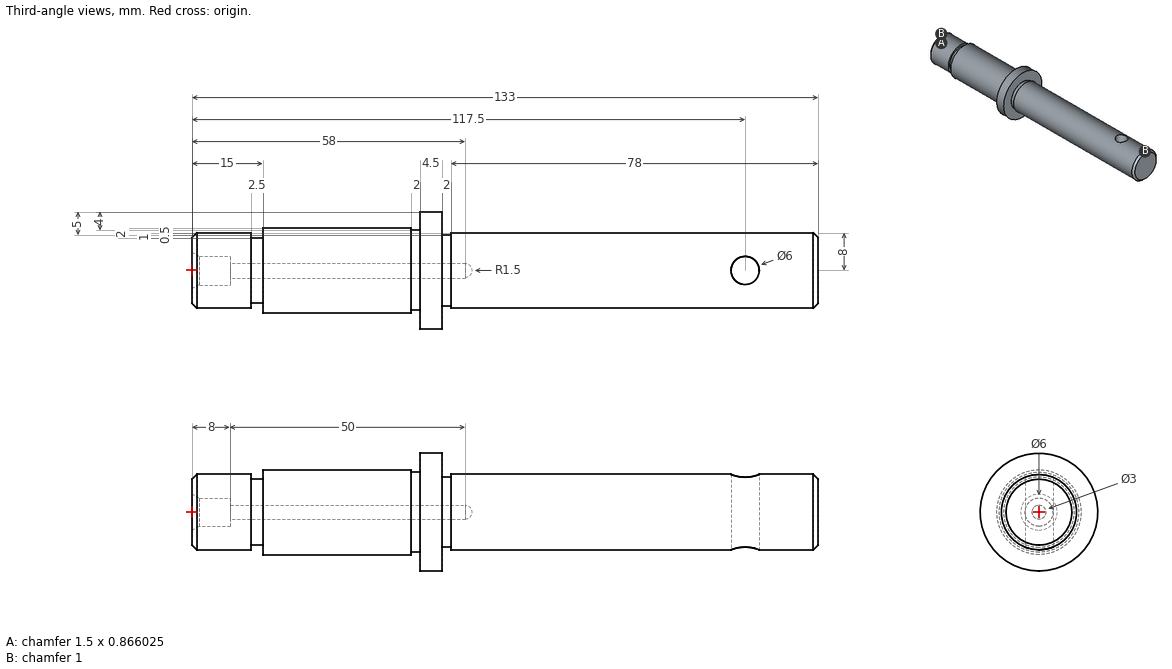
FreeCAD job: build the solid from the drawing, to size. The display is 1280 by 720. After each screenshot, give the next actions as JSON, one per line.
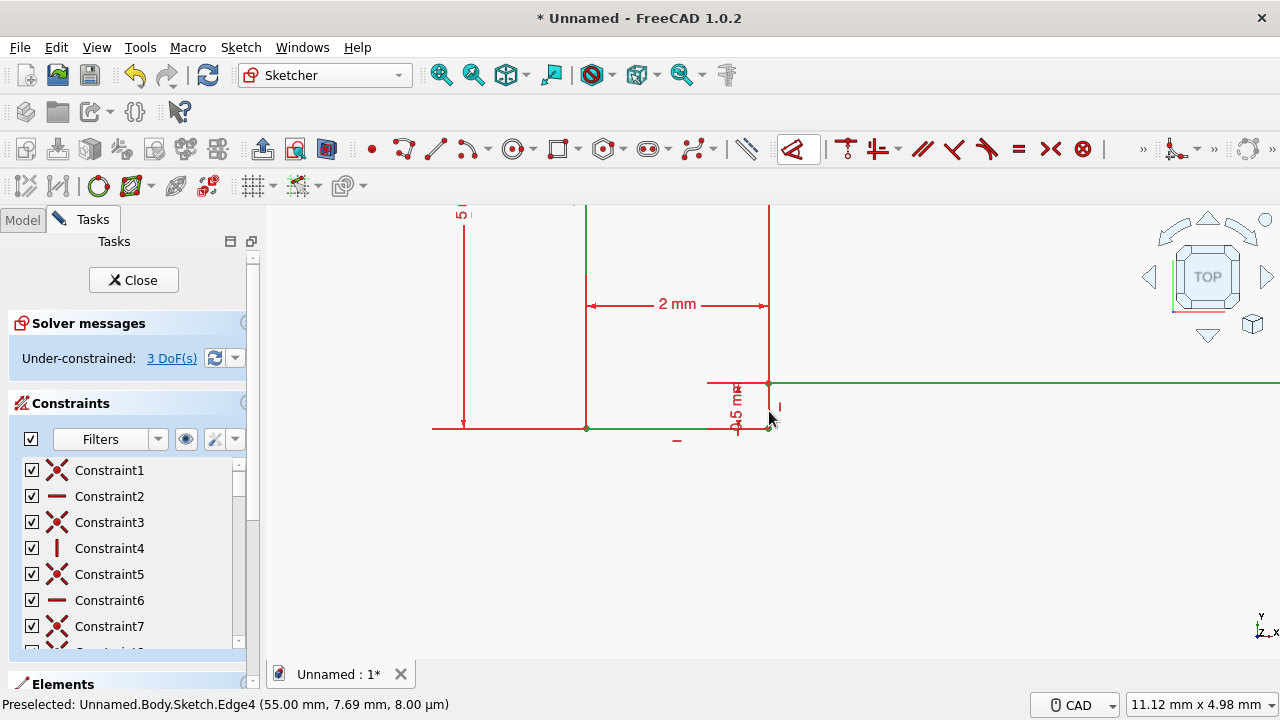
{"action": "scroll", "coordinate": [646, 426], "scroll_direction": "down", "scroll_amount": 15}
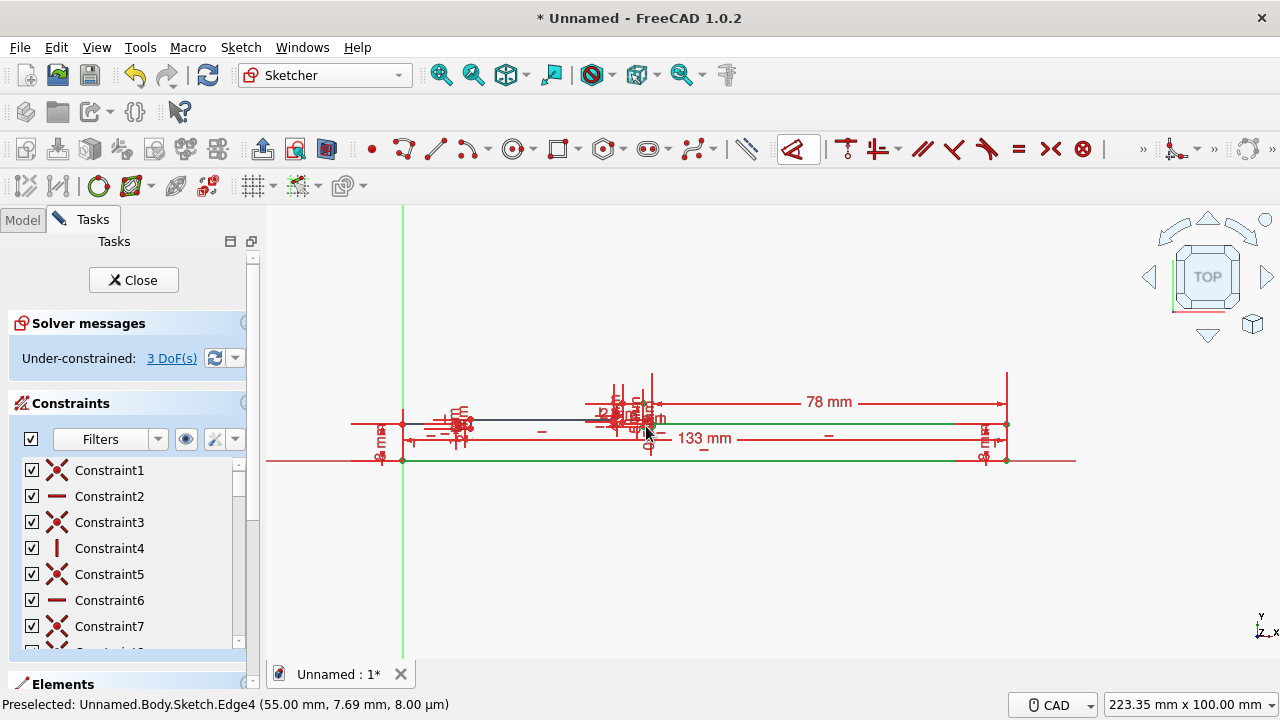
{"action": "scroll", "coordinate": [637, 404], "scroll_direction": "up", "scroll_amount": 5}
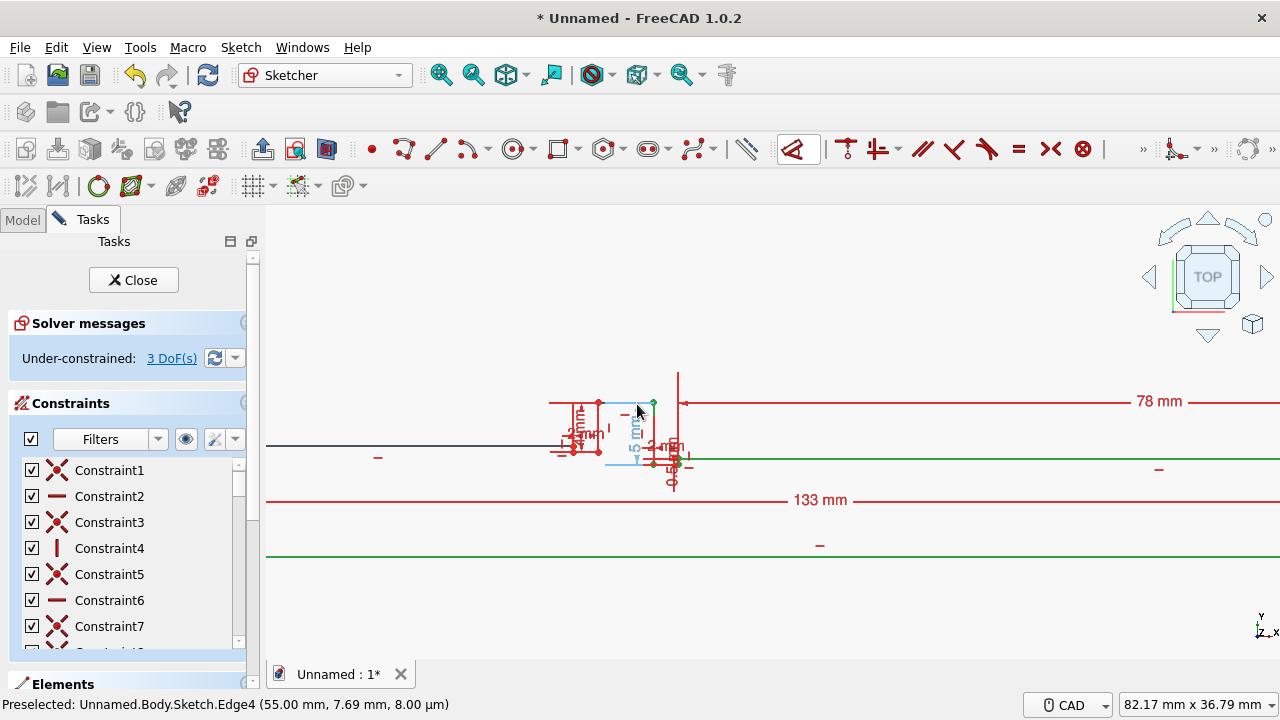
{"action": "left_click", "coordinate": [637, 403]}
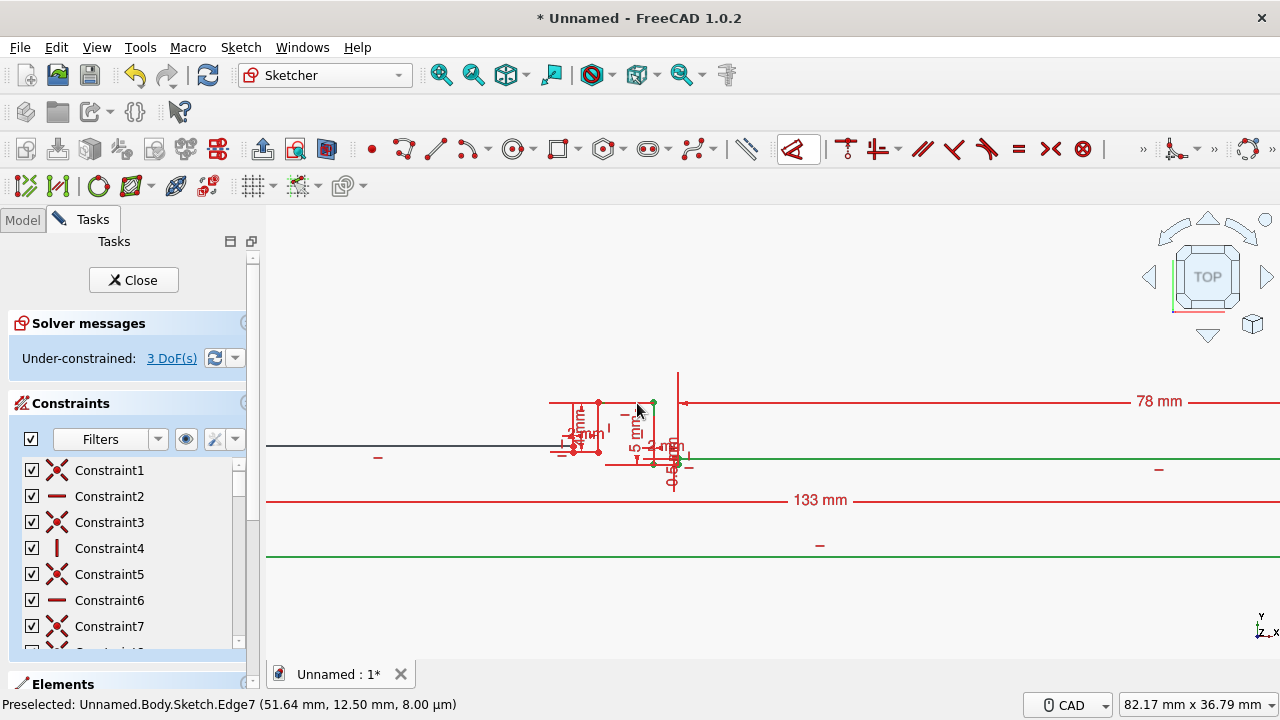
{"action": "key", "text": "l"}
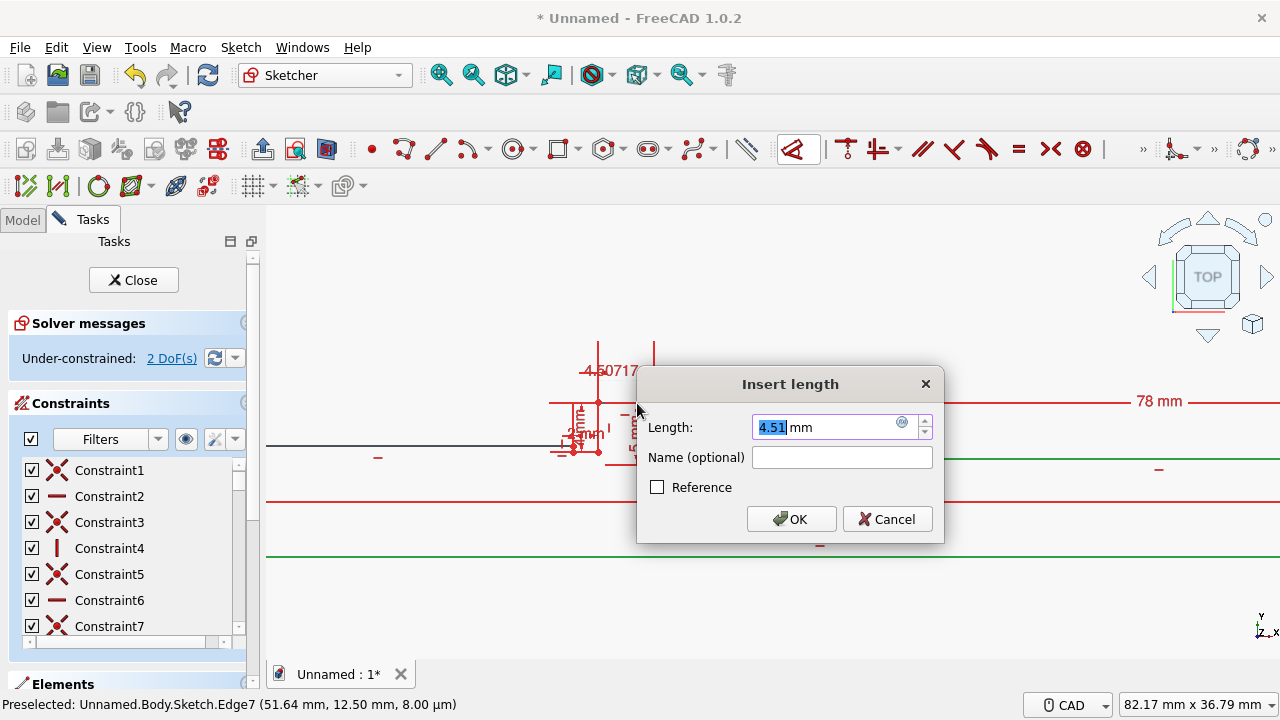
{"action": "type", "text": "4.5"}
{"action": "key", "text": "Return"}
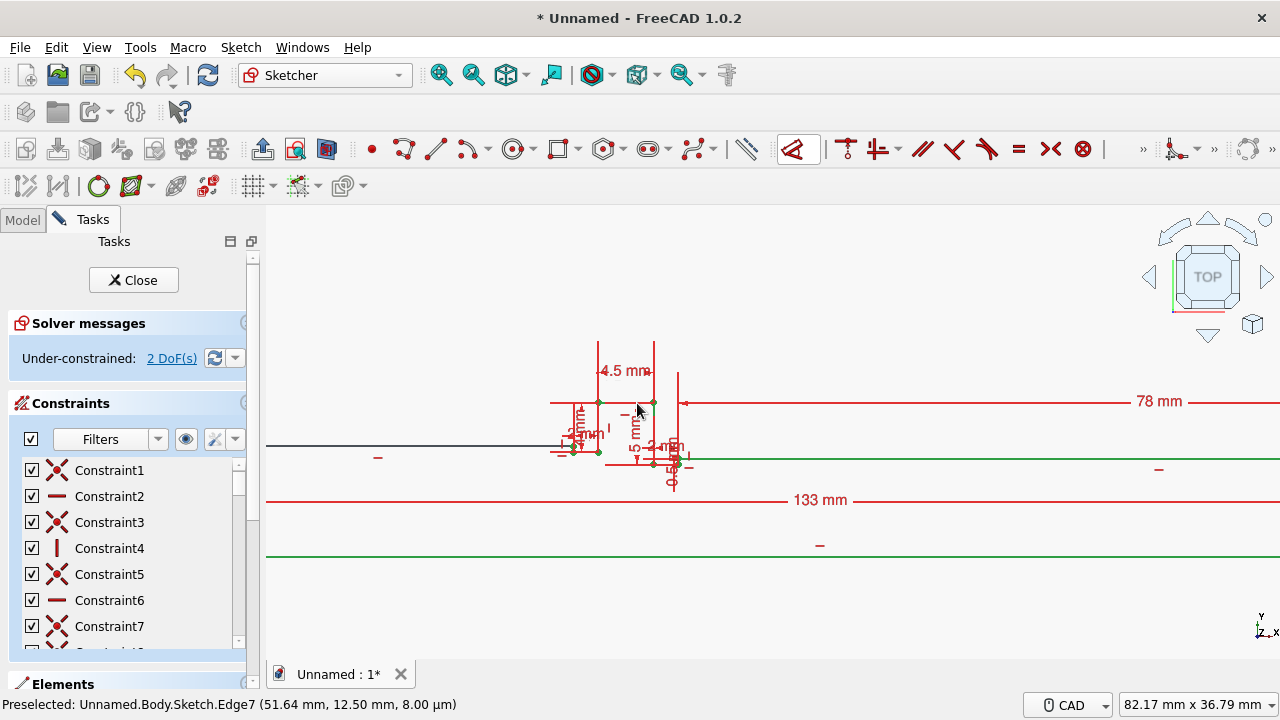
{"action": "scroll", "coordinate": [637, 404], "scroll_direction": "down", "scroll_amount": 5}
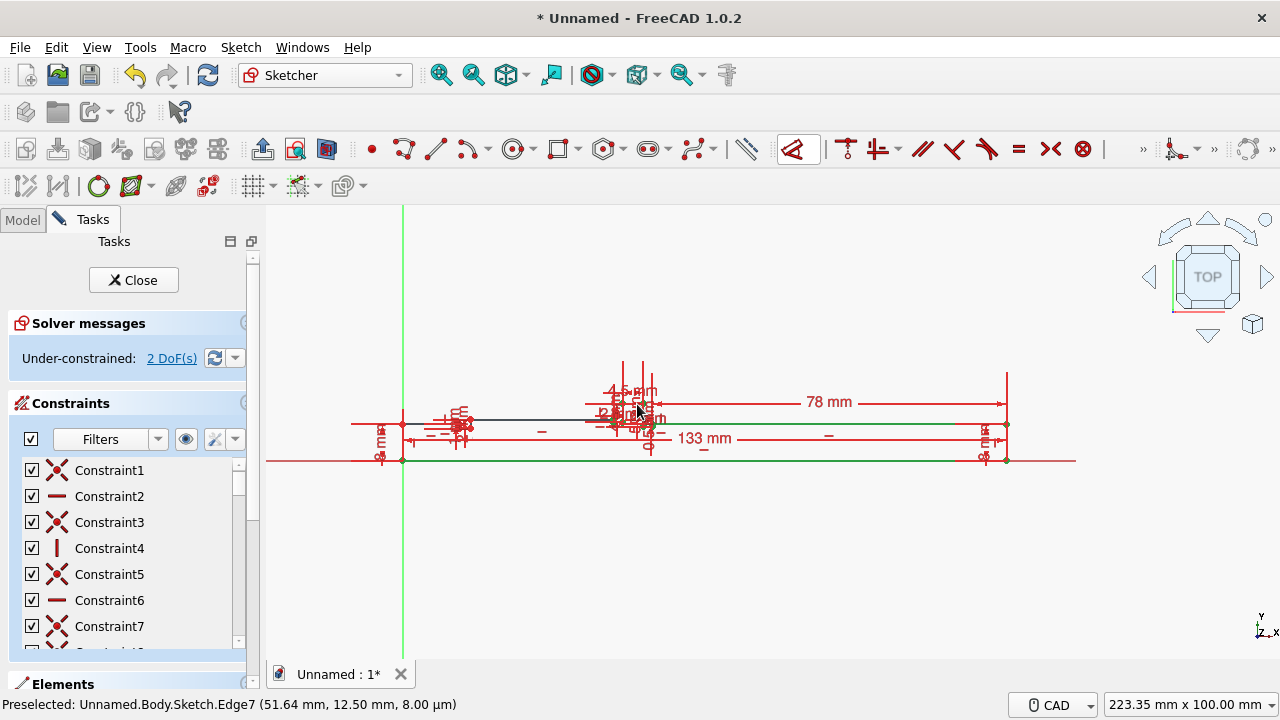
{"action": "scroll", "coordinate": [467, 429], "scroll_direction": "up", "scroll_amount": 7}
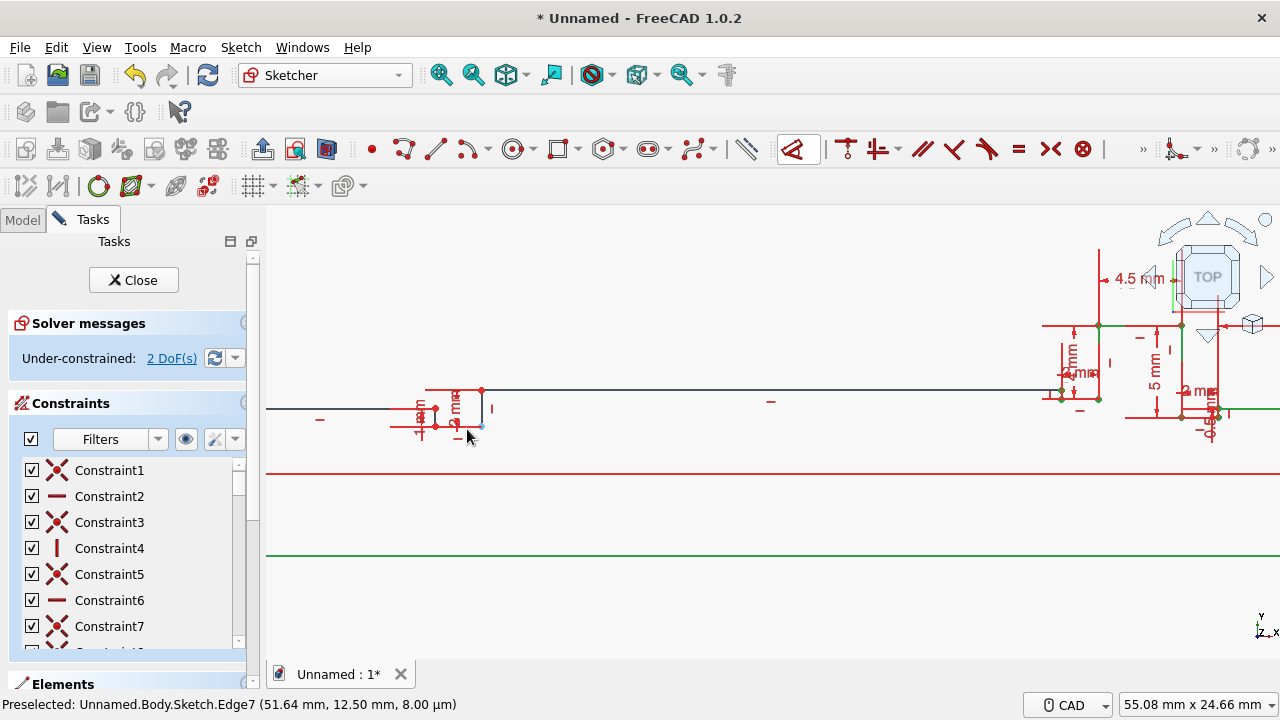
{"action": "left_click", "coordinate": [468, 427]}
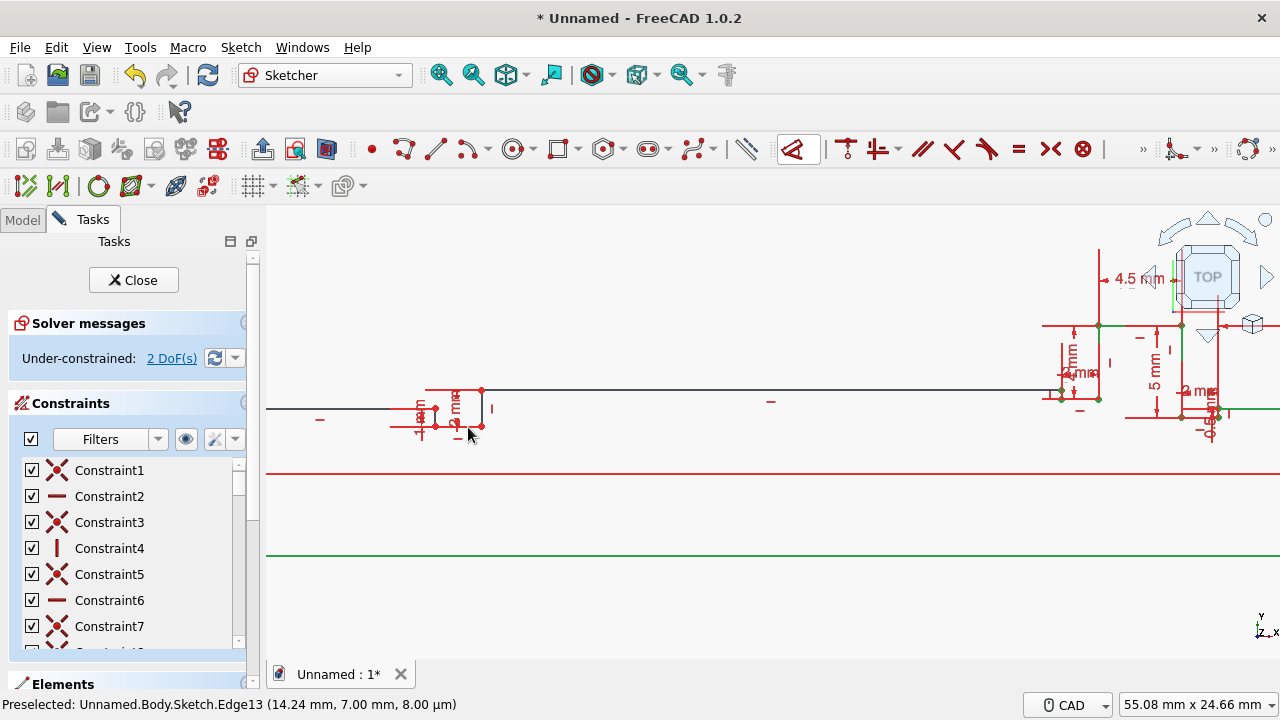
{"action": "left_click", "coordinate": [814, 150]}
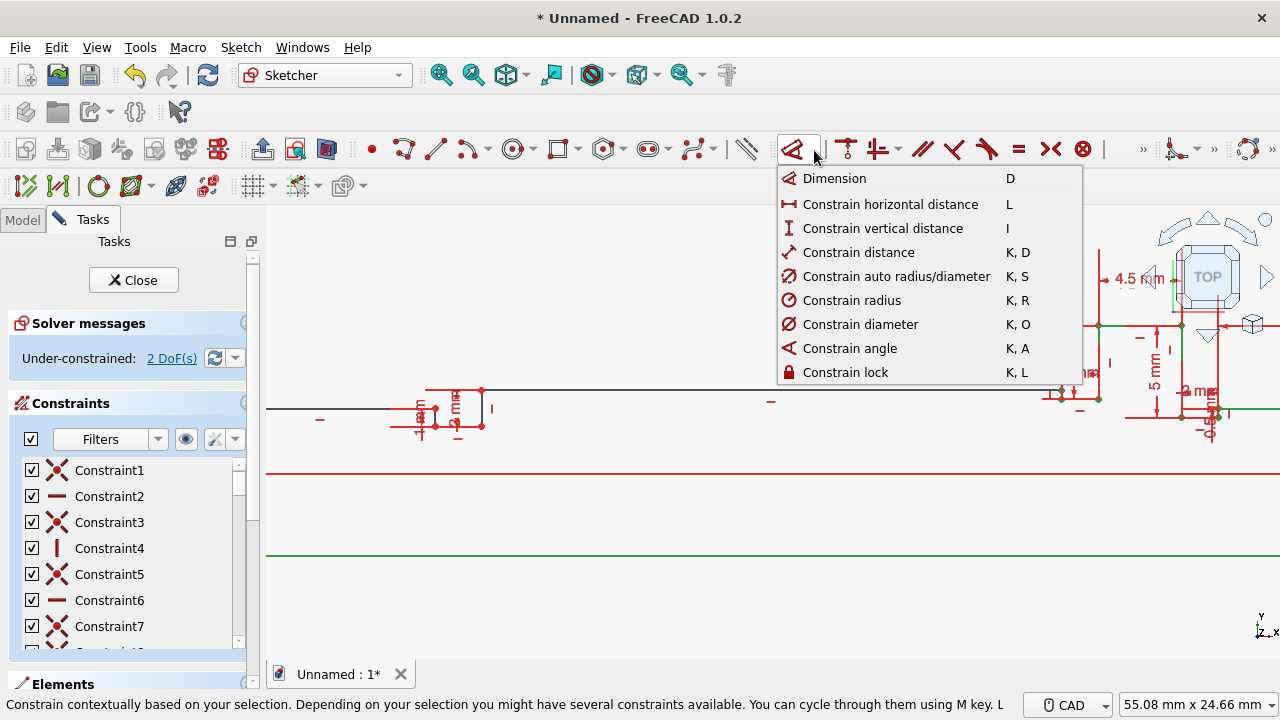
{"action": "left_click", "coordinate": [930, 204]}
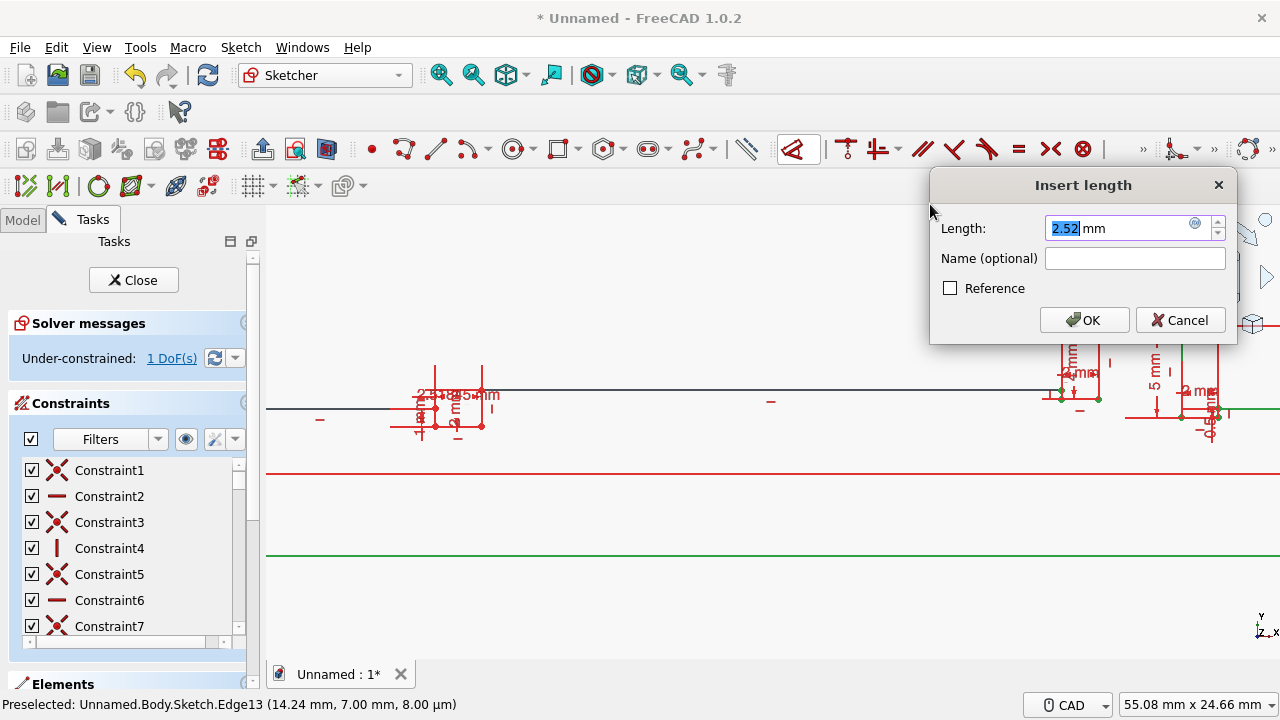
{"action": "type", "text": "2.5"}
{"action": "key", "text": "Return"}